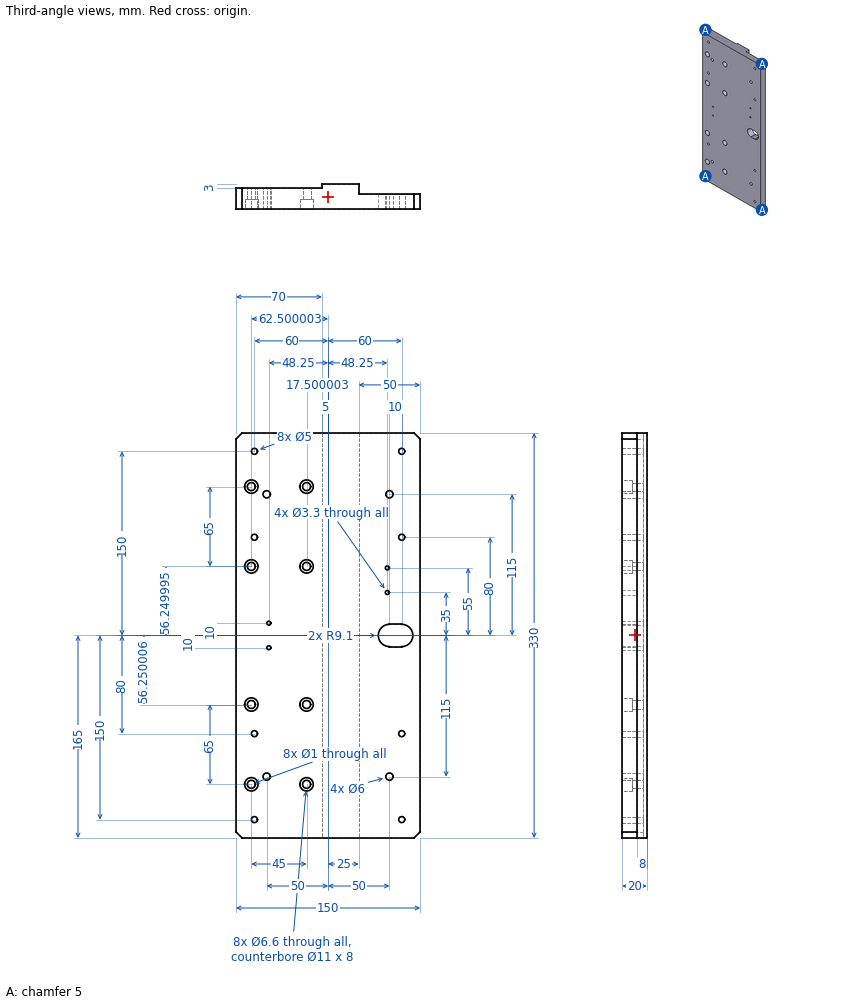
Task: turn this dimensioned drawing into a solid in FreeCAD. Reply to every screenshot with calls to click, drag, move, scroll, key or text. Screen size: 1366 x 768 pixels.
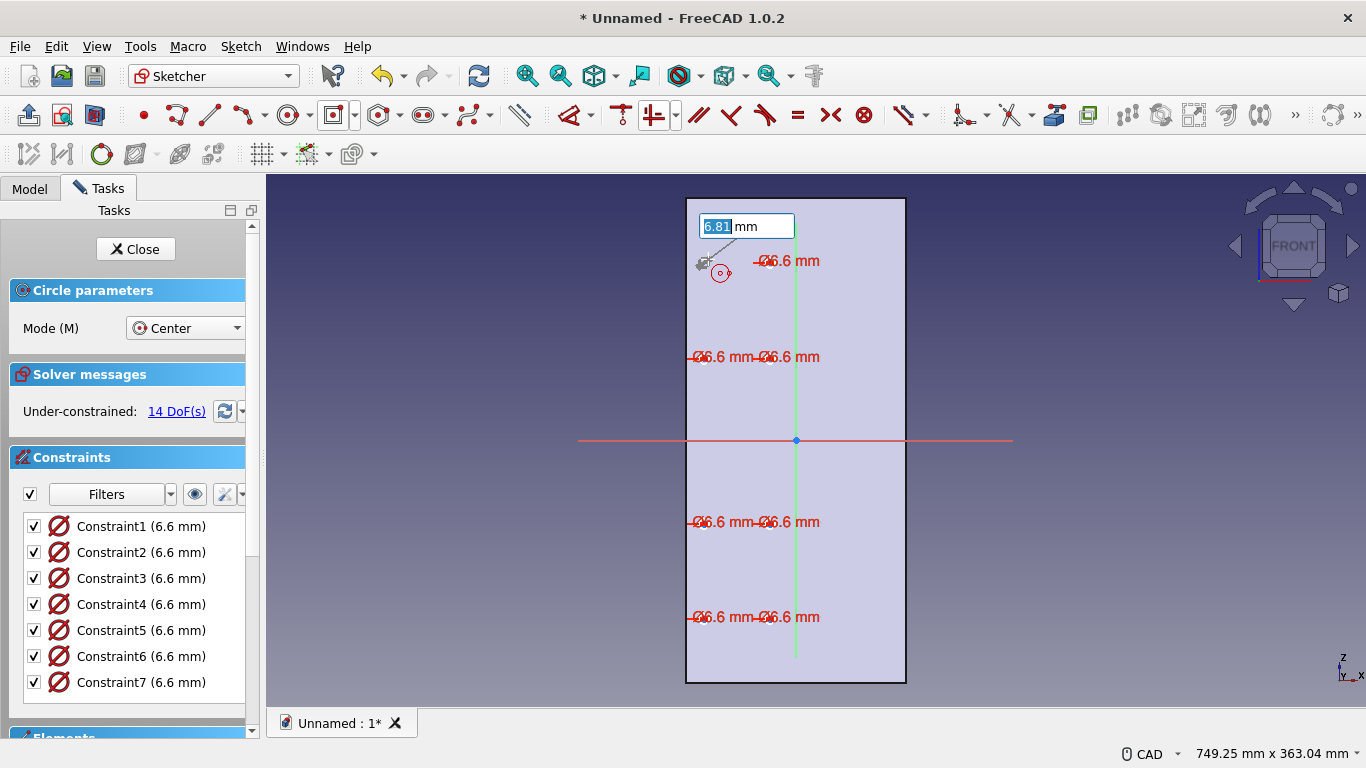
text(6.6)
key(Return)
key(Escape)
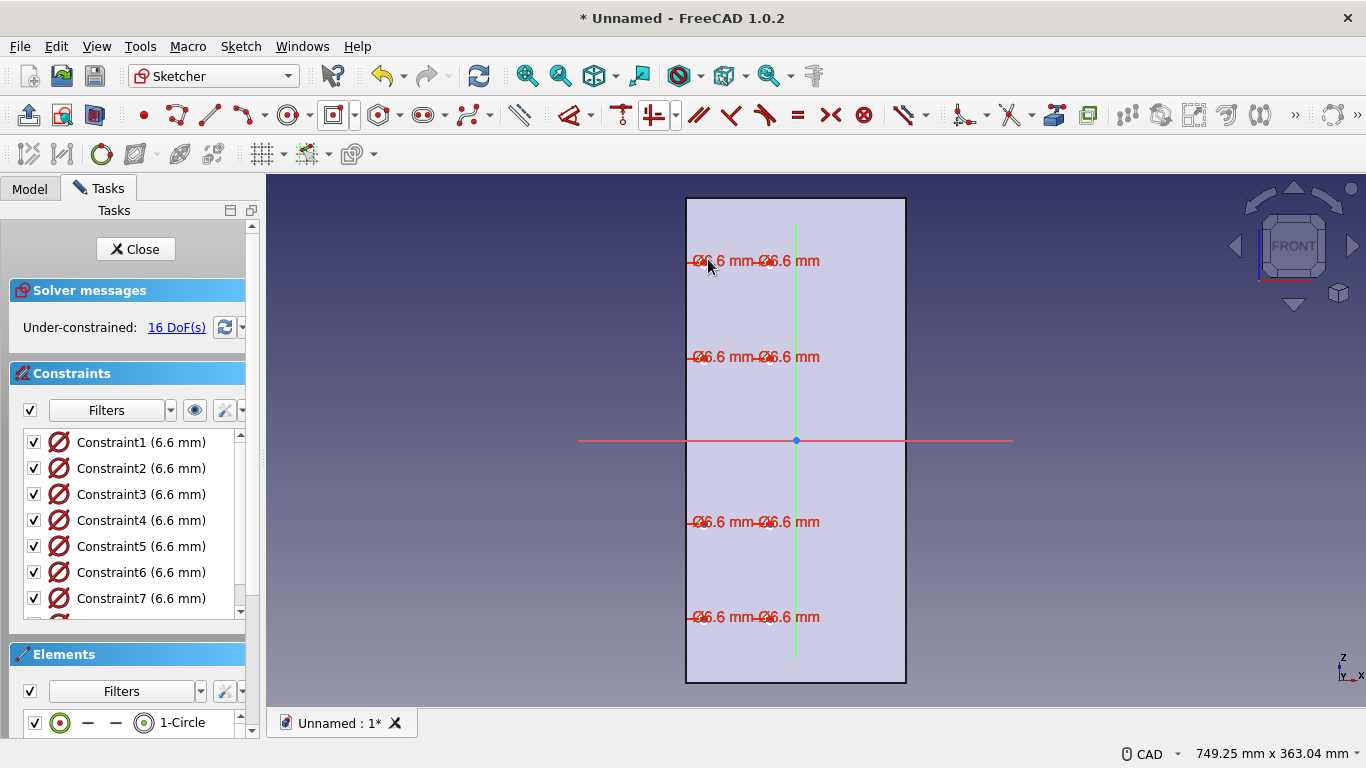
click(770, 619)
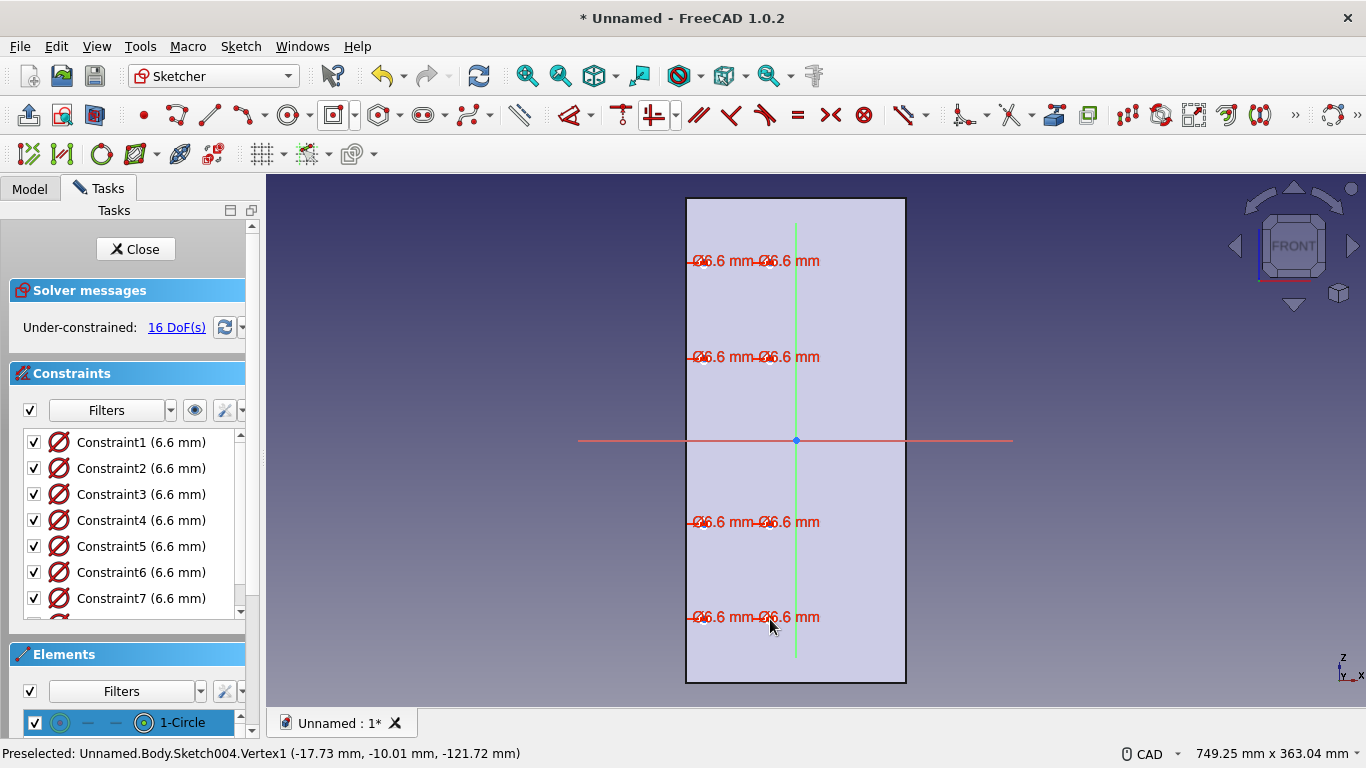
click(704, 619)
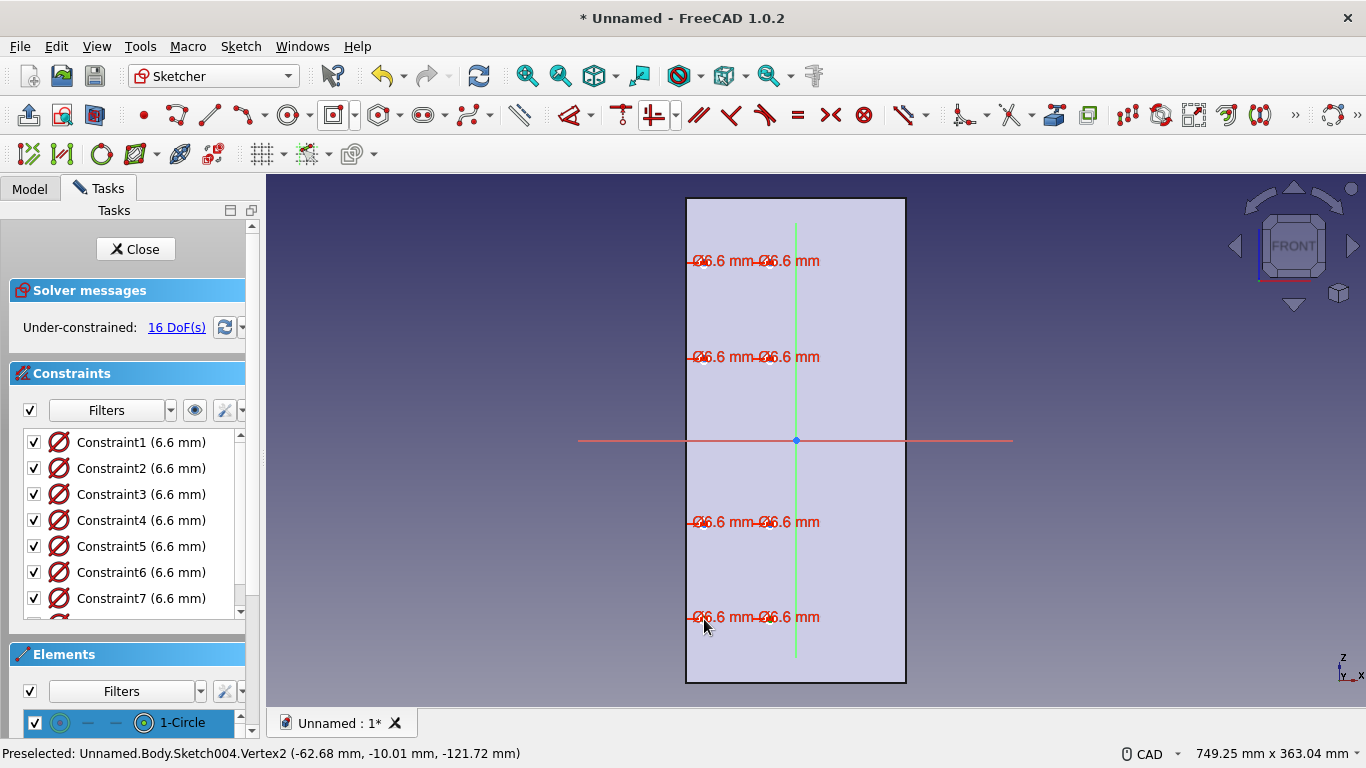
click(676, 116)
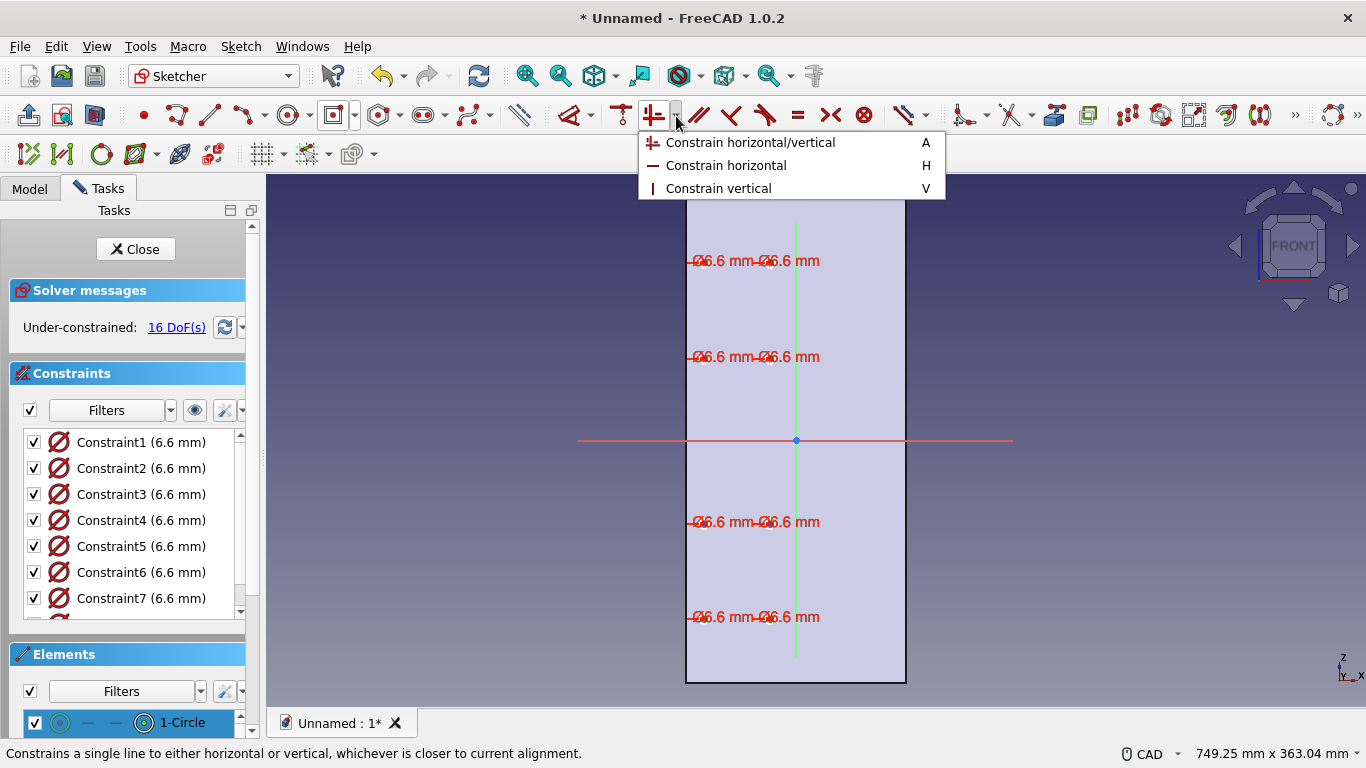
click(792, 166)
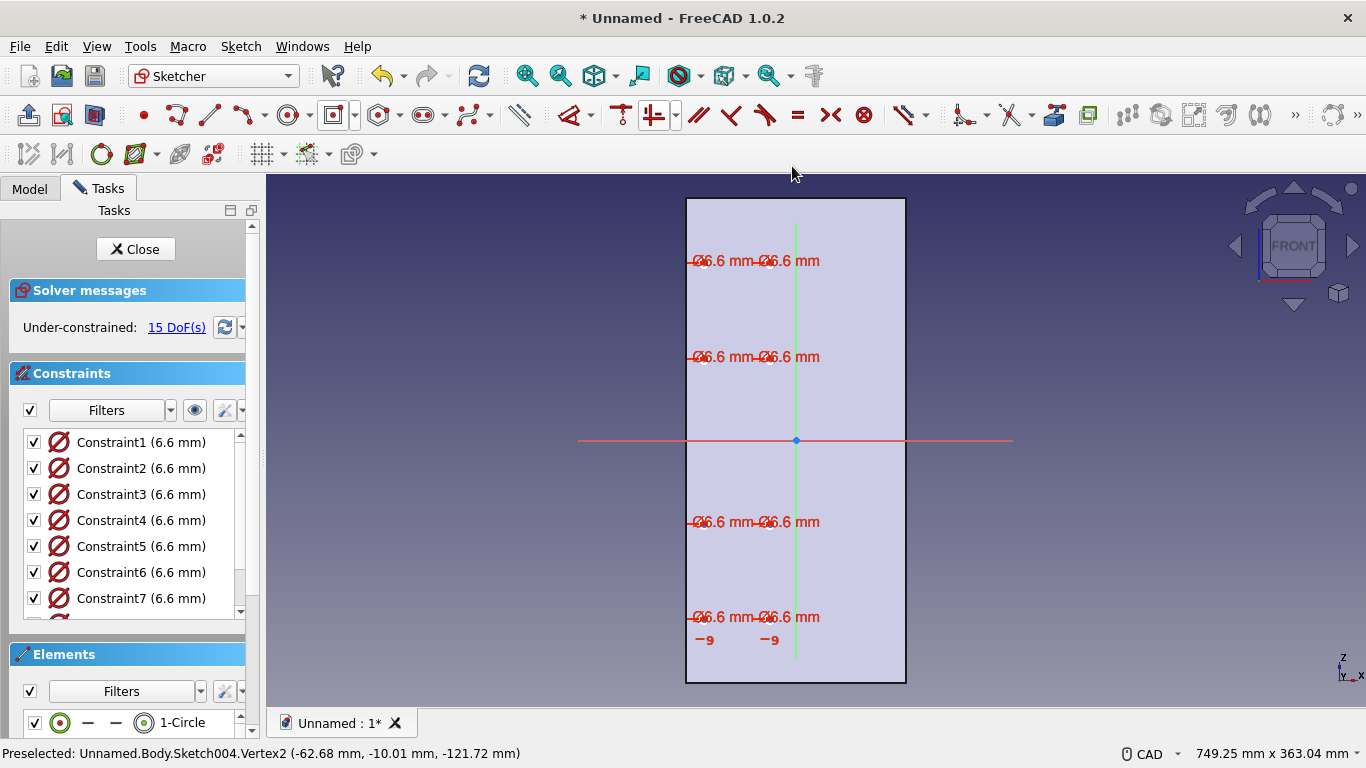
click(770, 619)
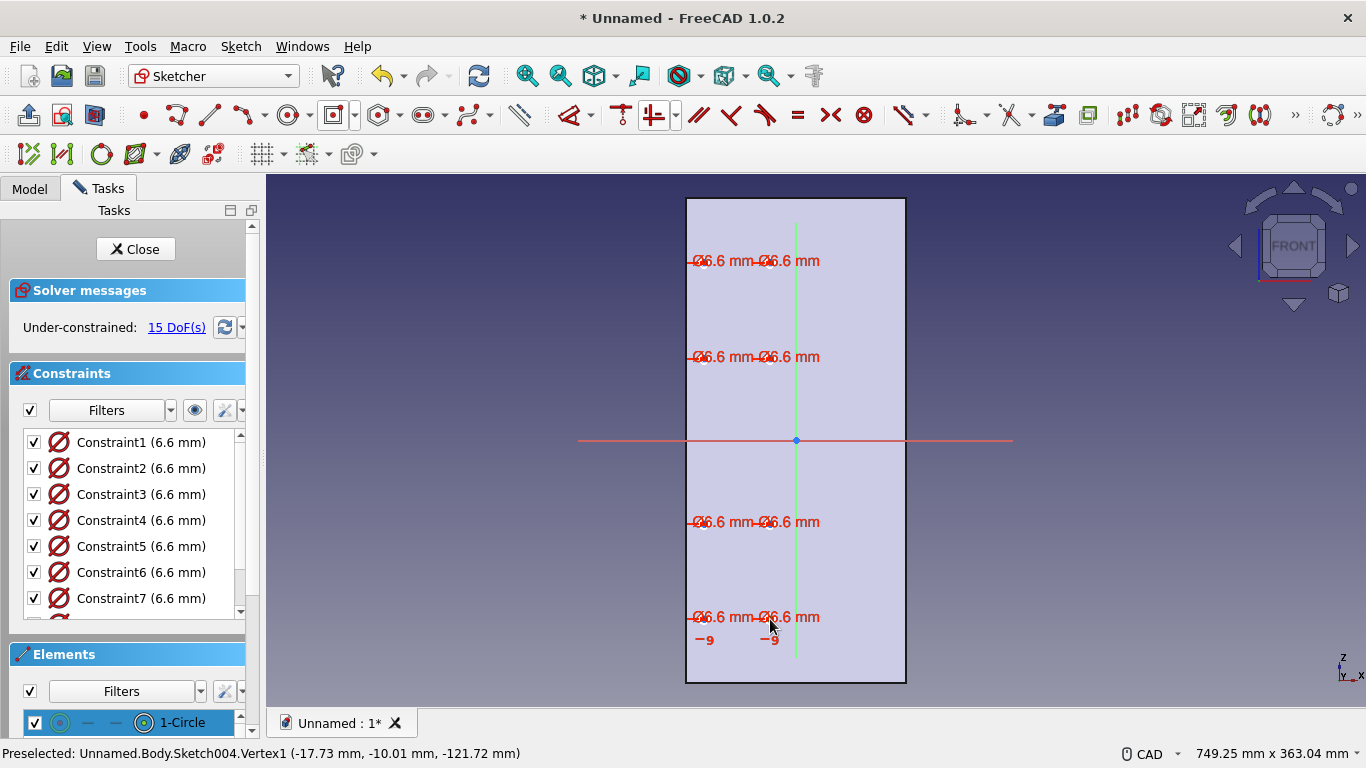
click(770, 524)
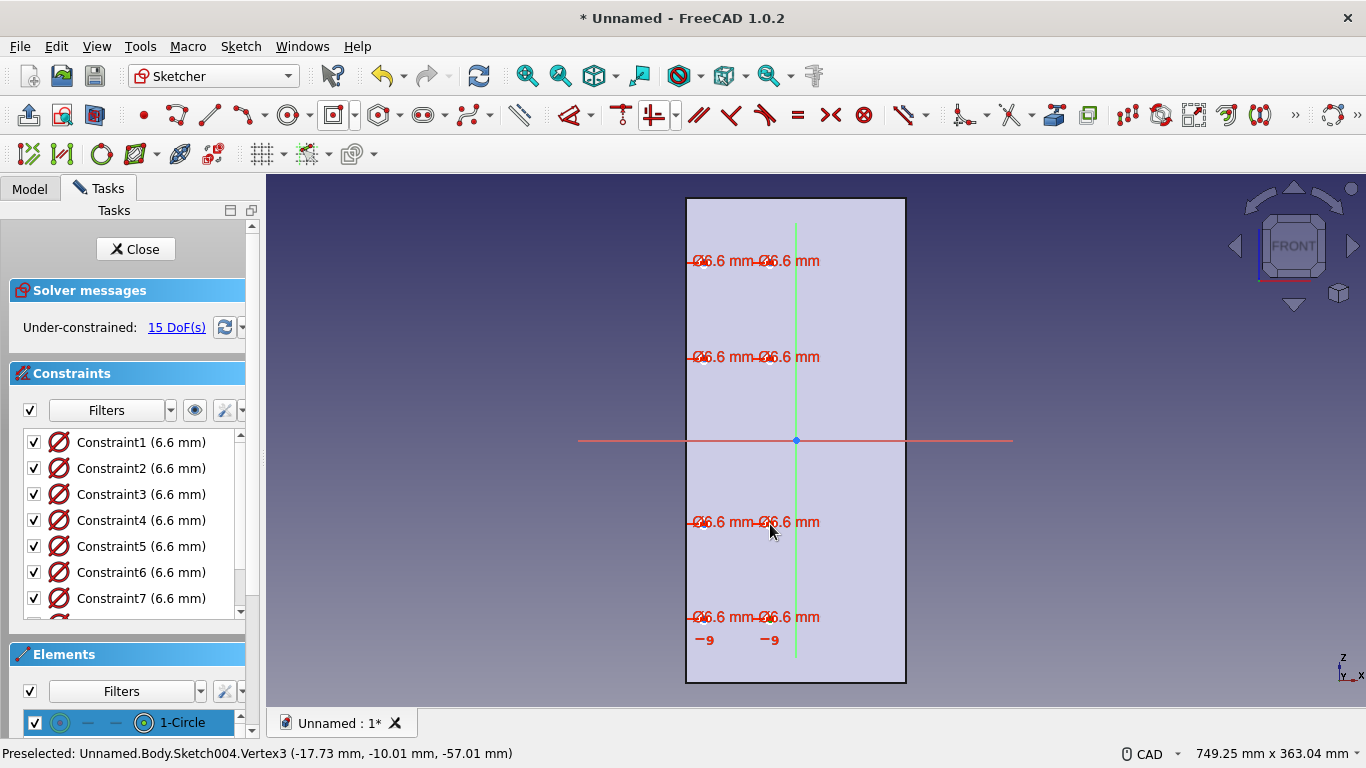
key(v)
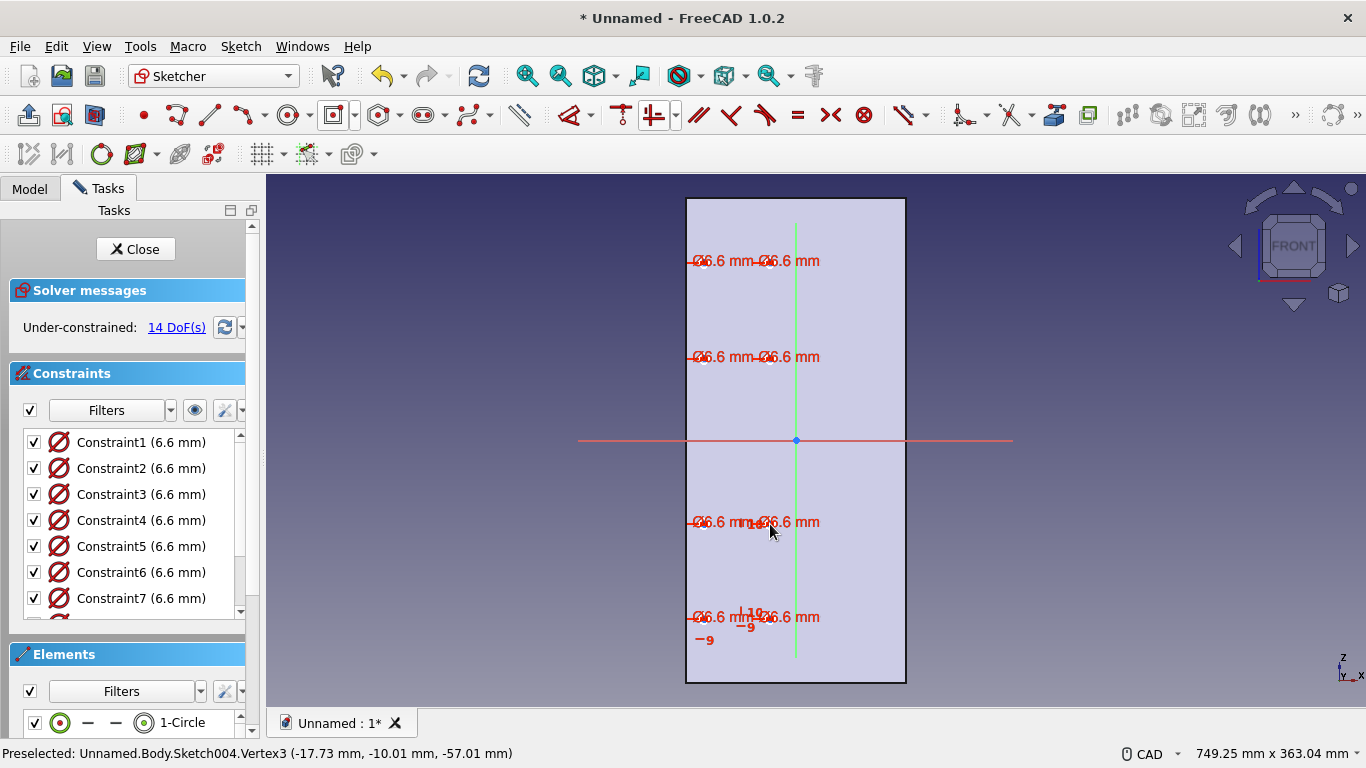
click(704, 619)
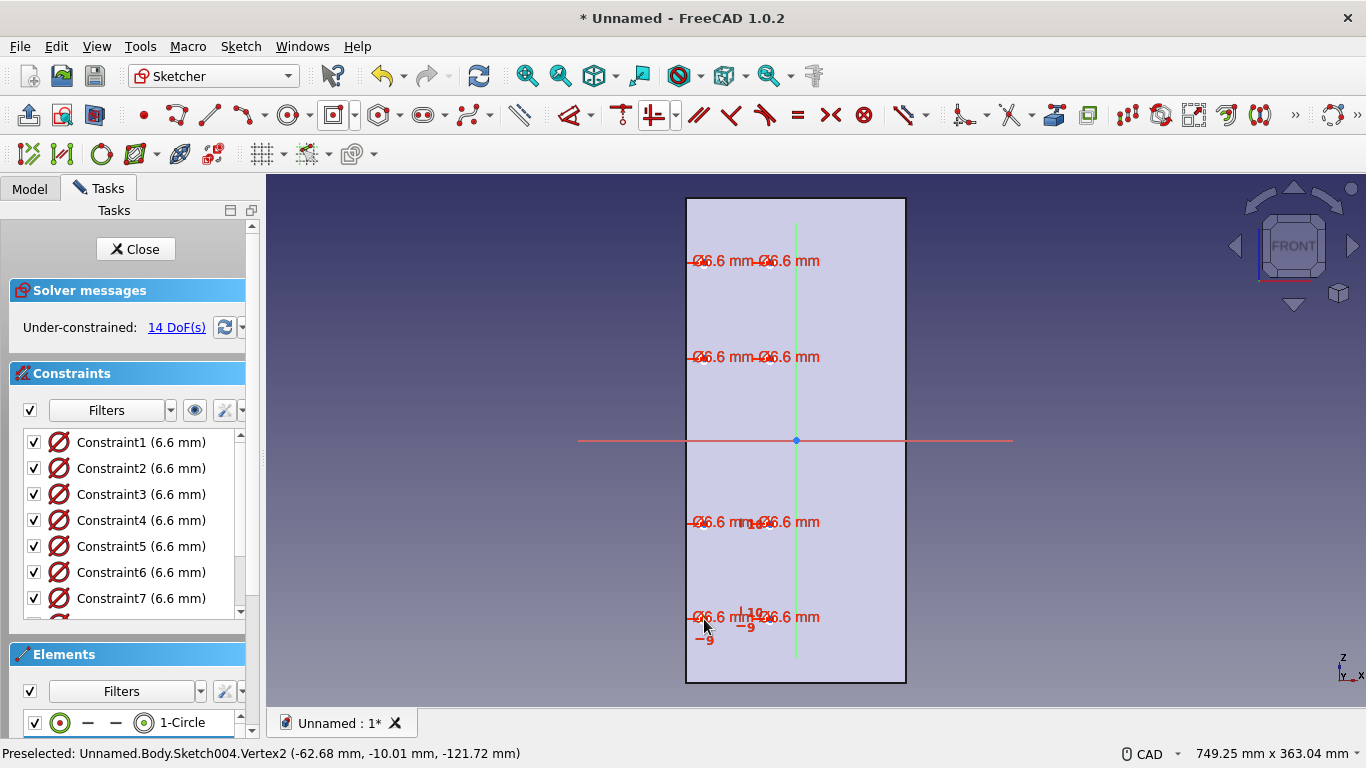
click(704, 524)